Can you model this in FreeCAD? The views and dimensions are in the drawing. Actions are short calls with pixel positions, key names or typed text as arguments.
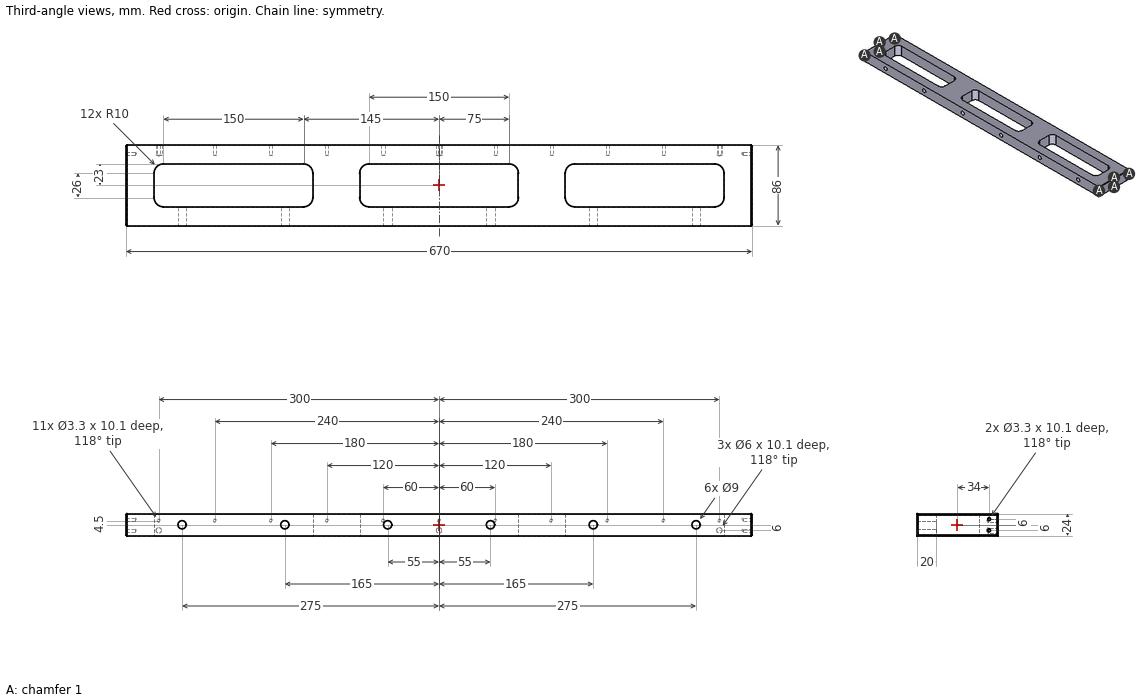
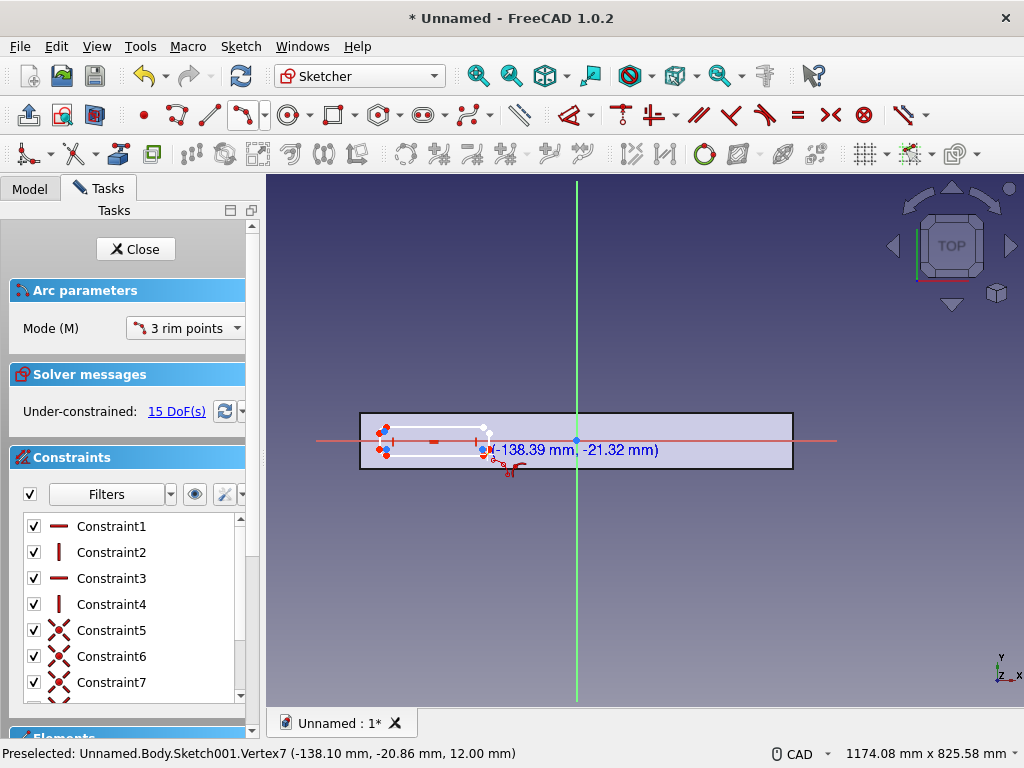
scroll(489, 432, up, 4)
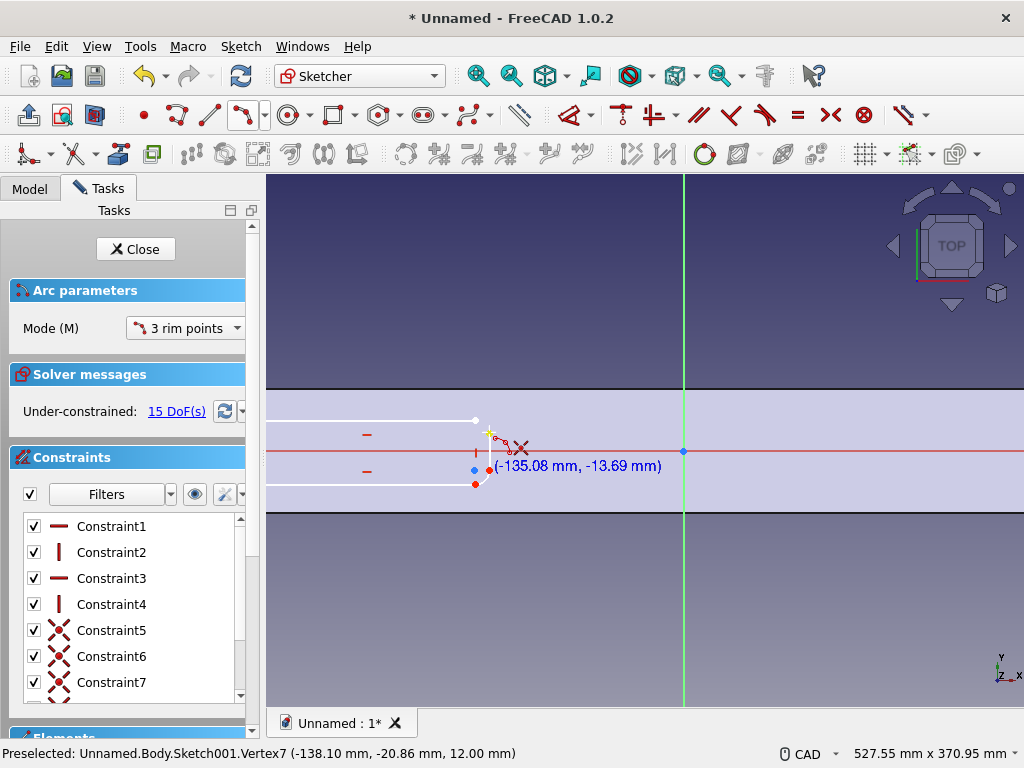
click(490, 434)
click(476, 421)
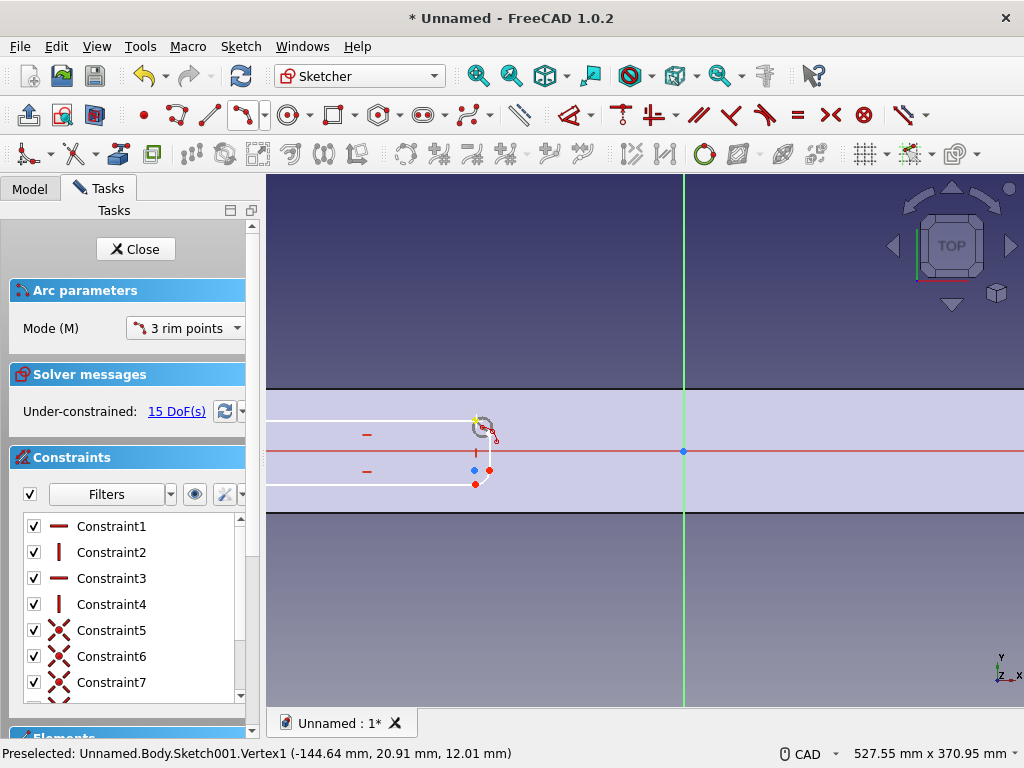
scroll(485, 422, up, 7)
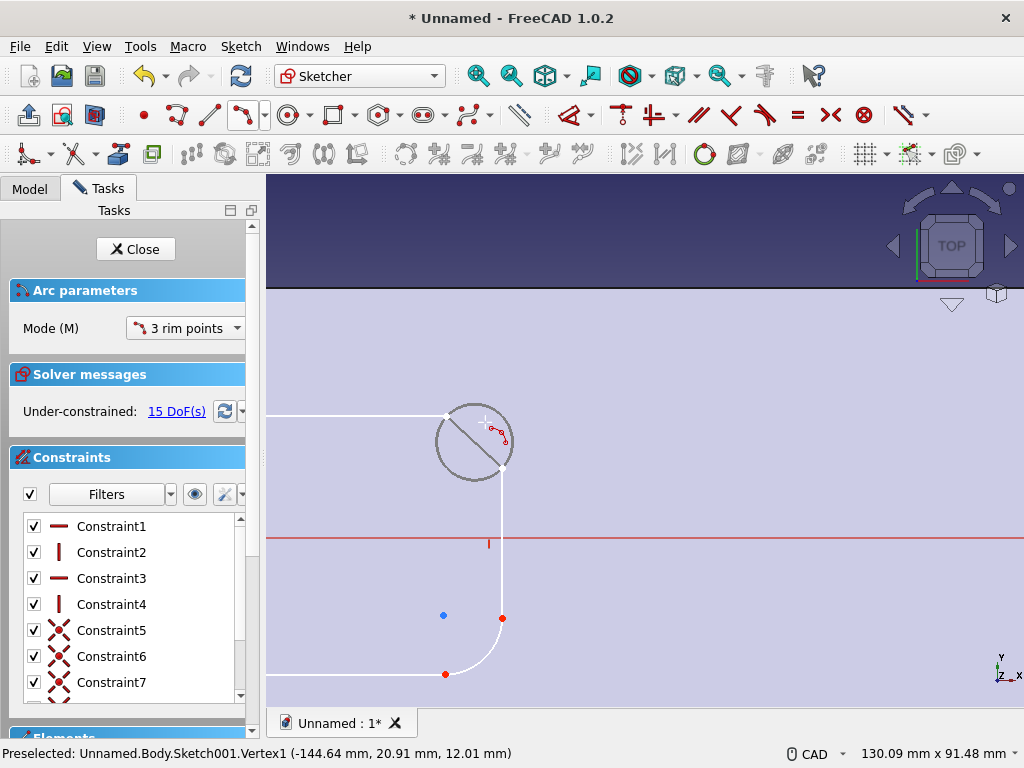
click(486, 421)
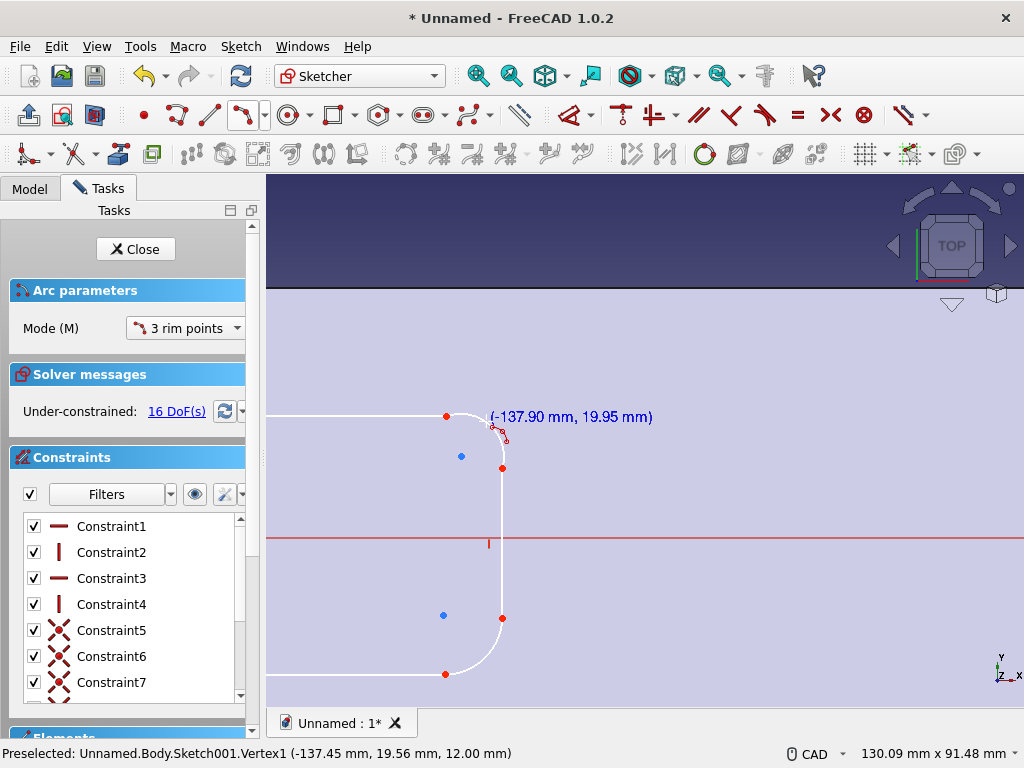
key(g)
key(l)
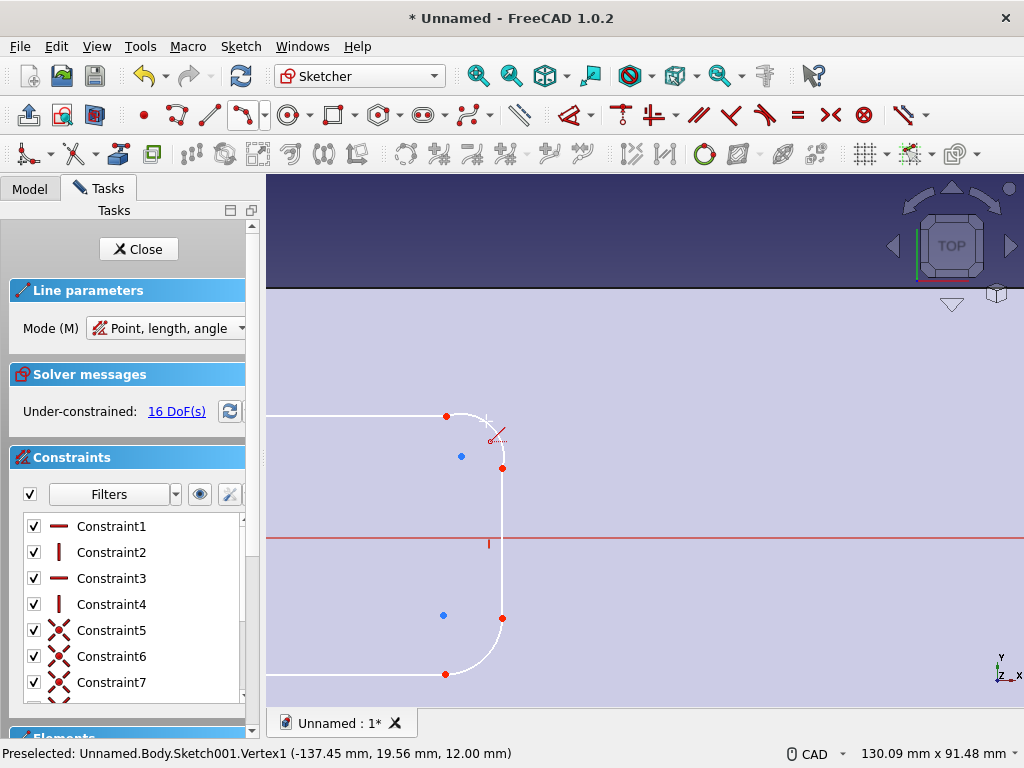
scroll(488, 428, down, 11)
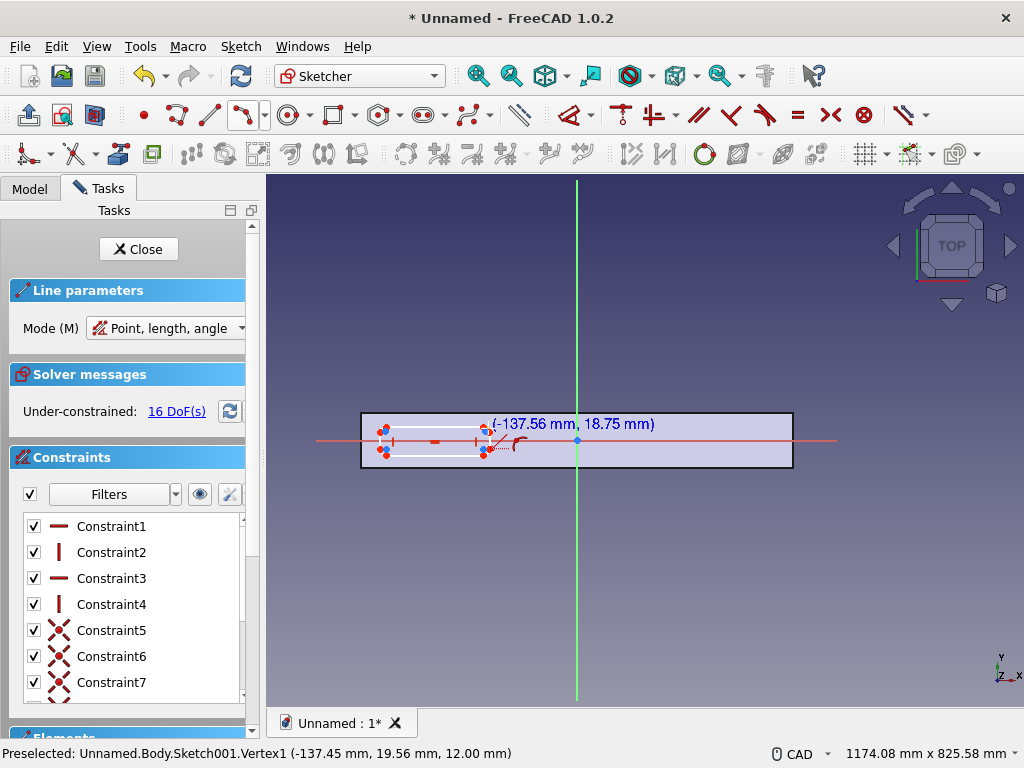
click(625, 426)
click(529, 426)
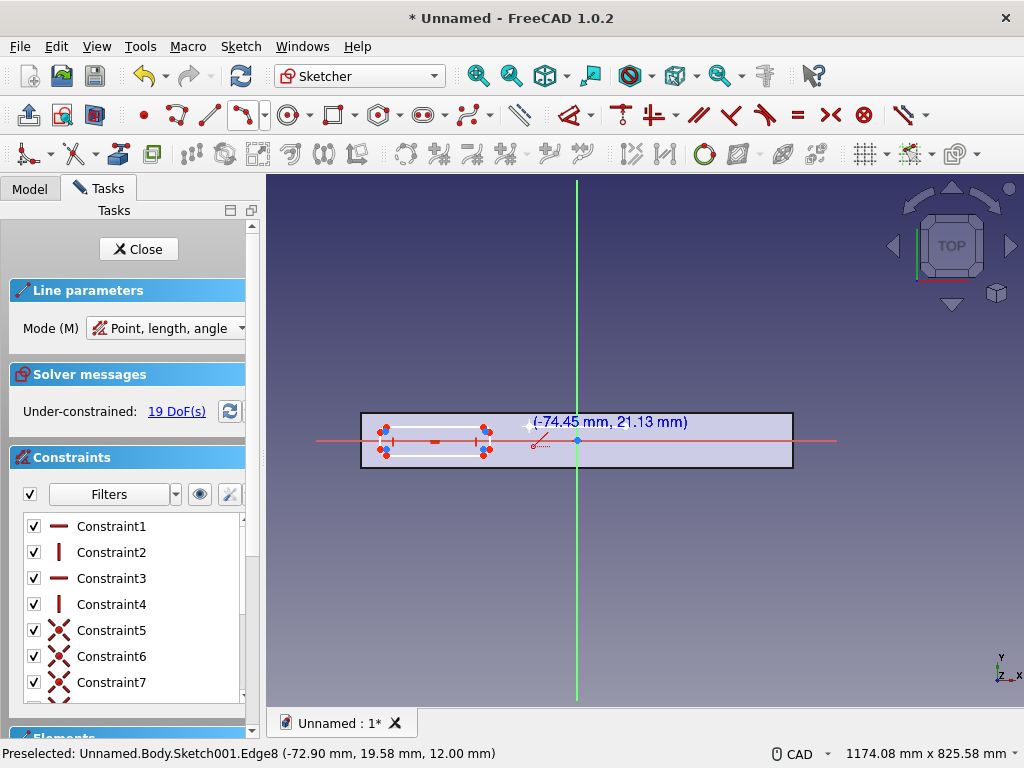
scroll(522, 432, up, 4)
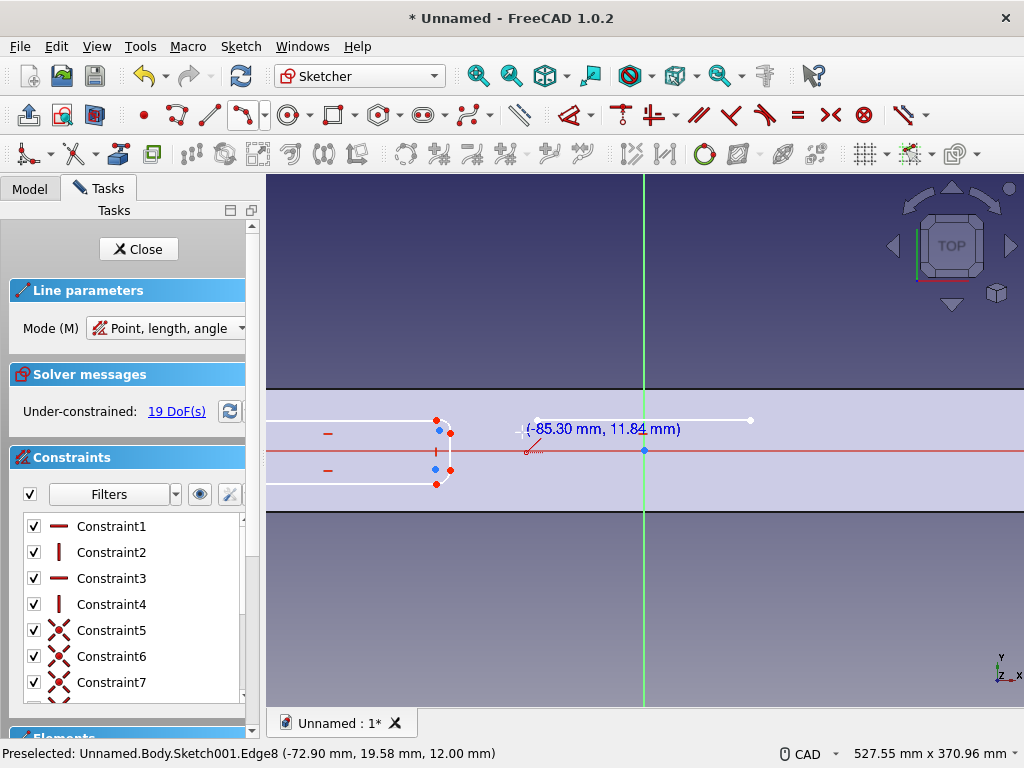
click(522, 432)
click(522, 469)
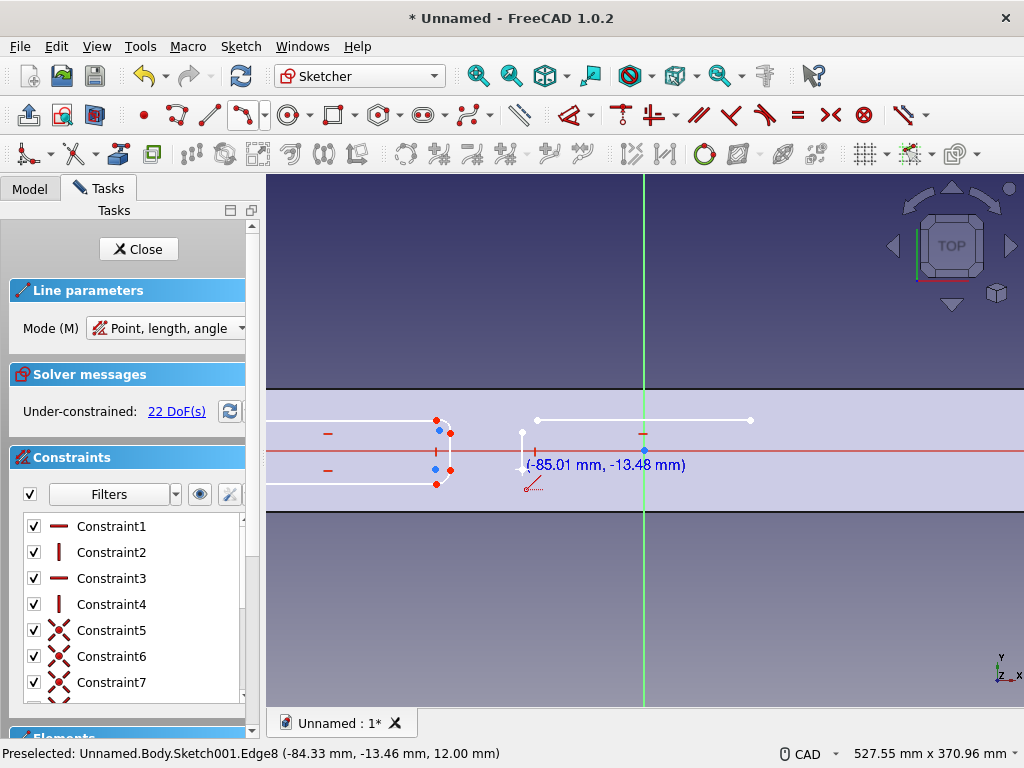
click(536, 484)
click(752, 484)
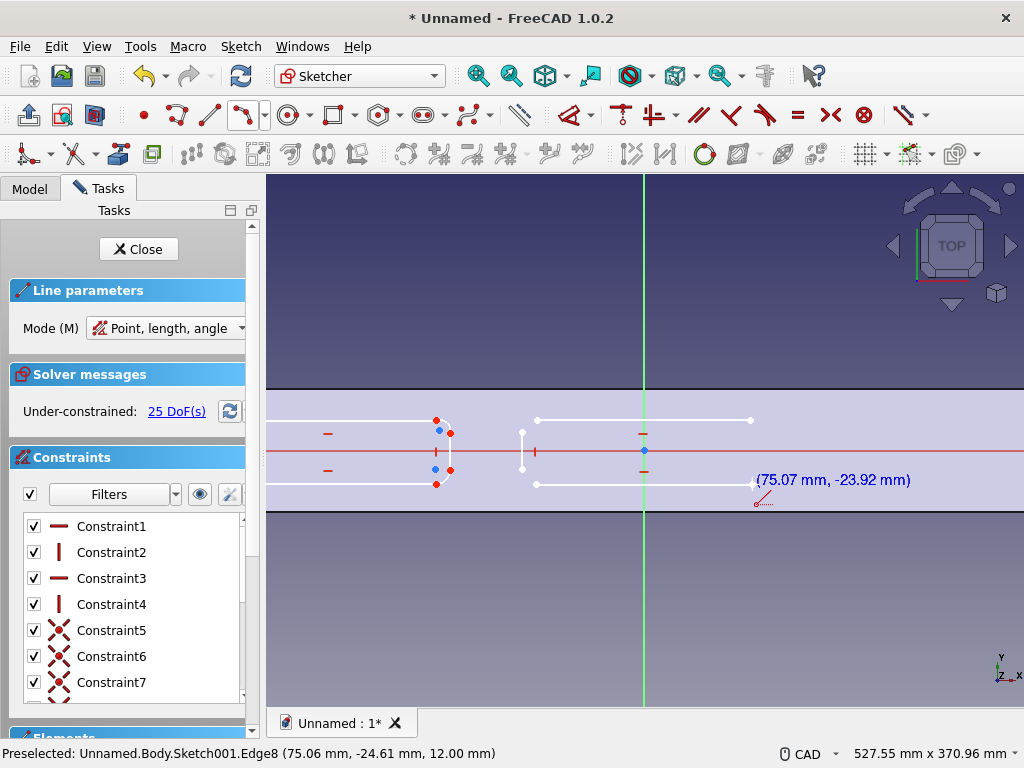
click(766, 469)
click(766, 432)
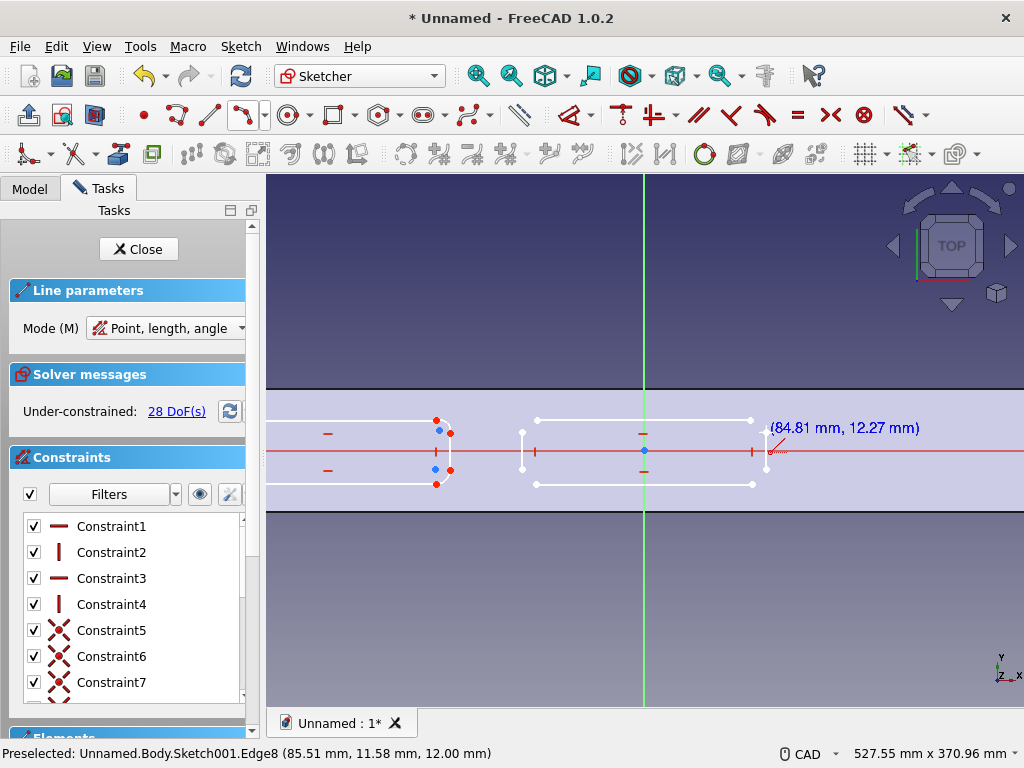
click(242, 116)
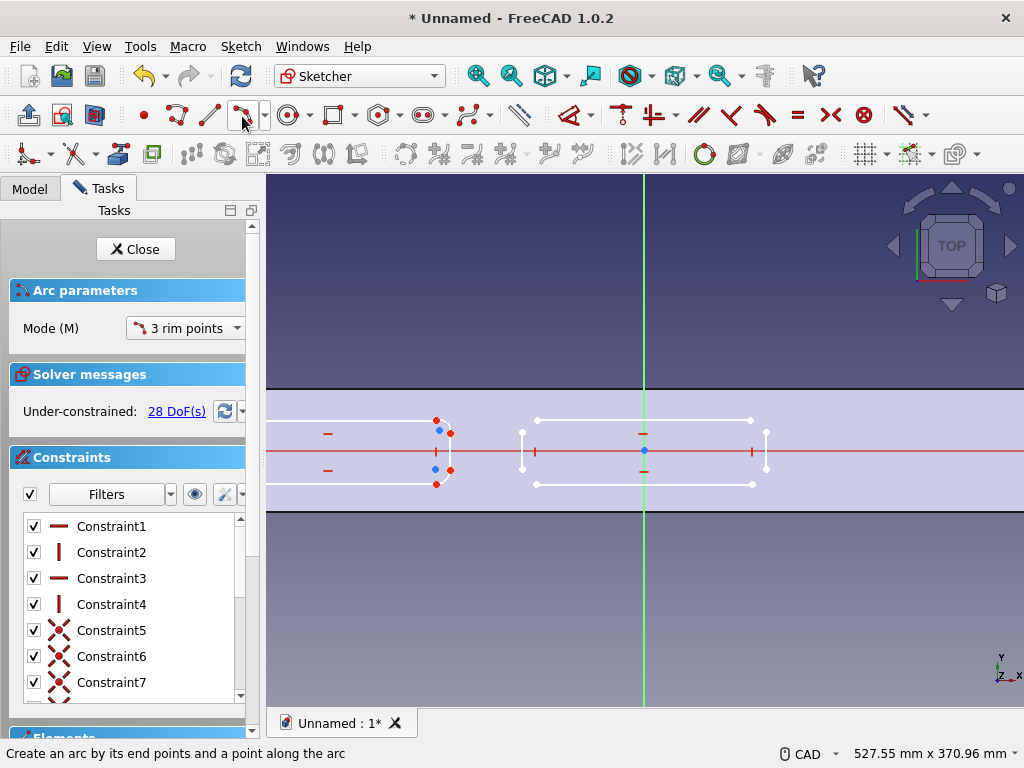
click(537, 420)
click(522, 433)